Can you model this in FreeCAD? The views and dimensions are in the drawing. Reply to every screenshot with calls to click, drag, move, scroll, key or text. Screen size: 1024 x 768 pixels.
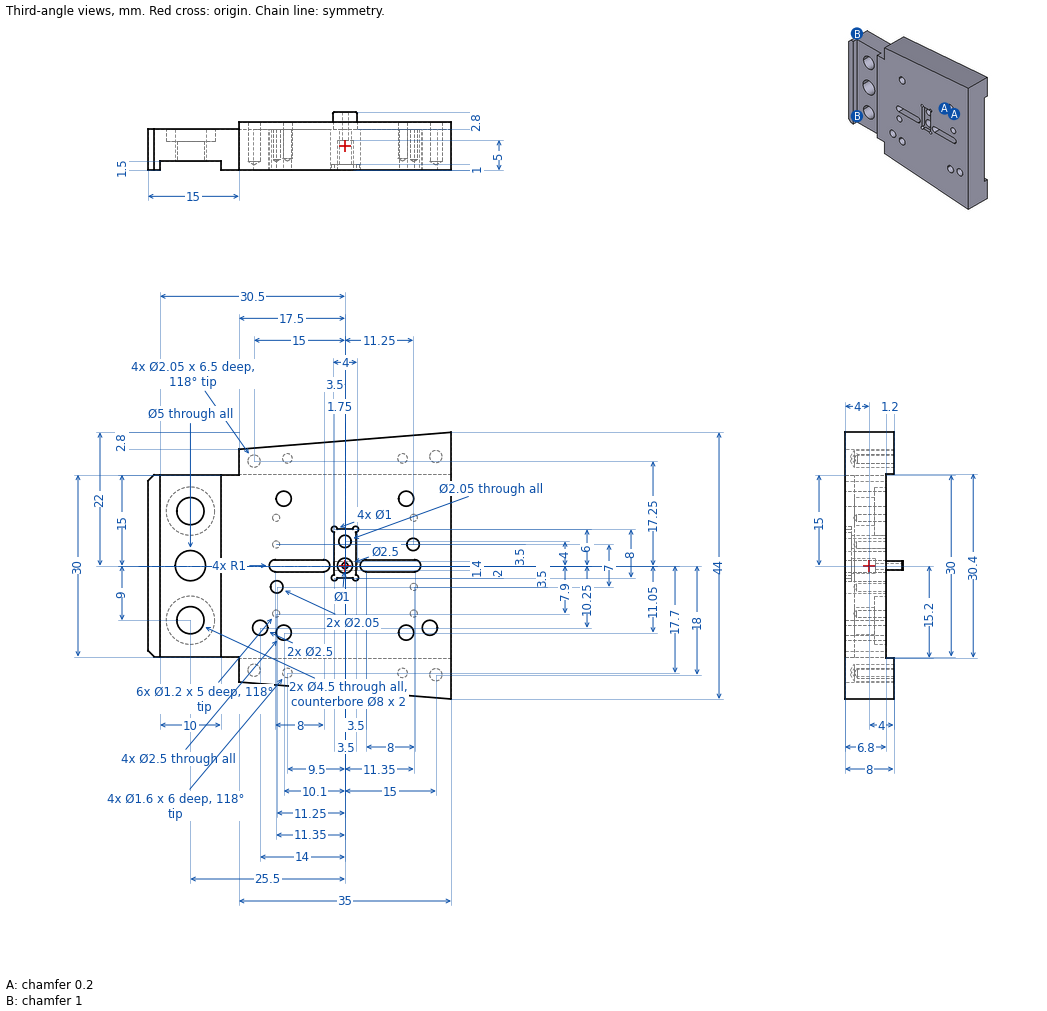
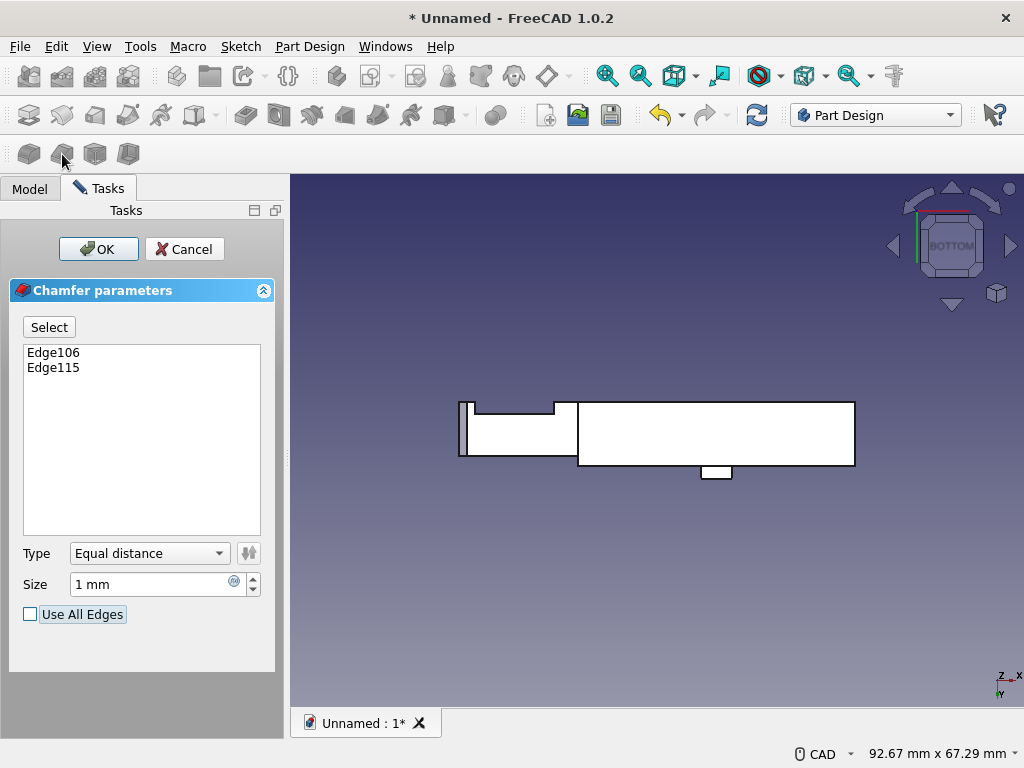
click(99, 249)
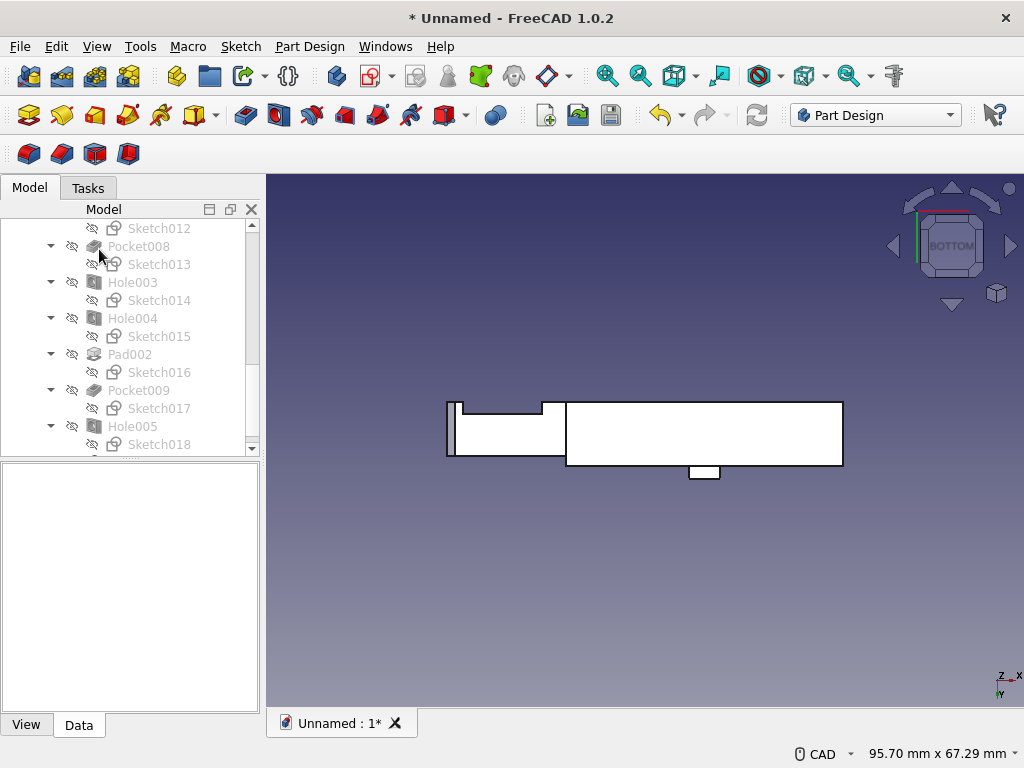
key(4)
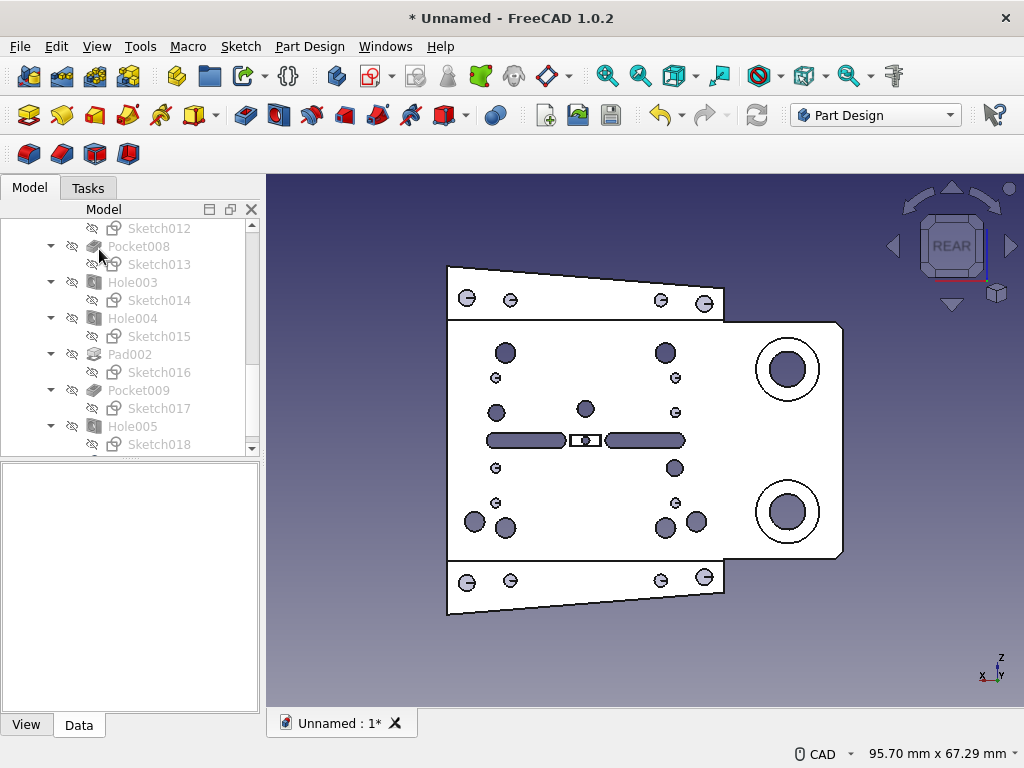
click(588, 508)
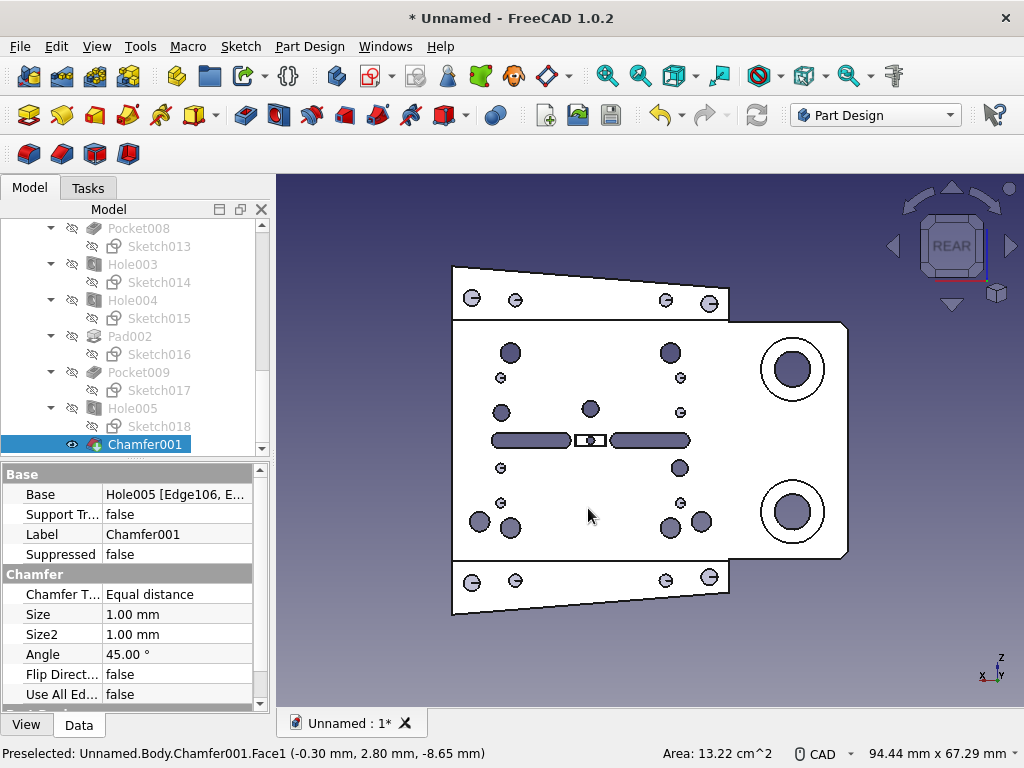
click(370, 76)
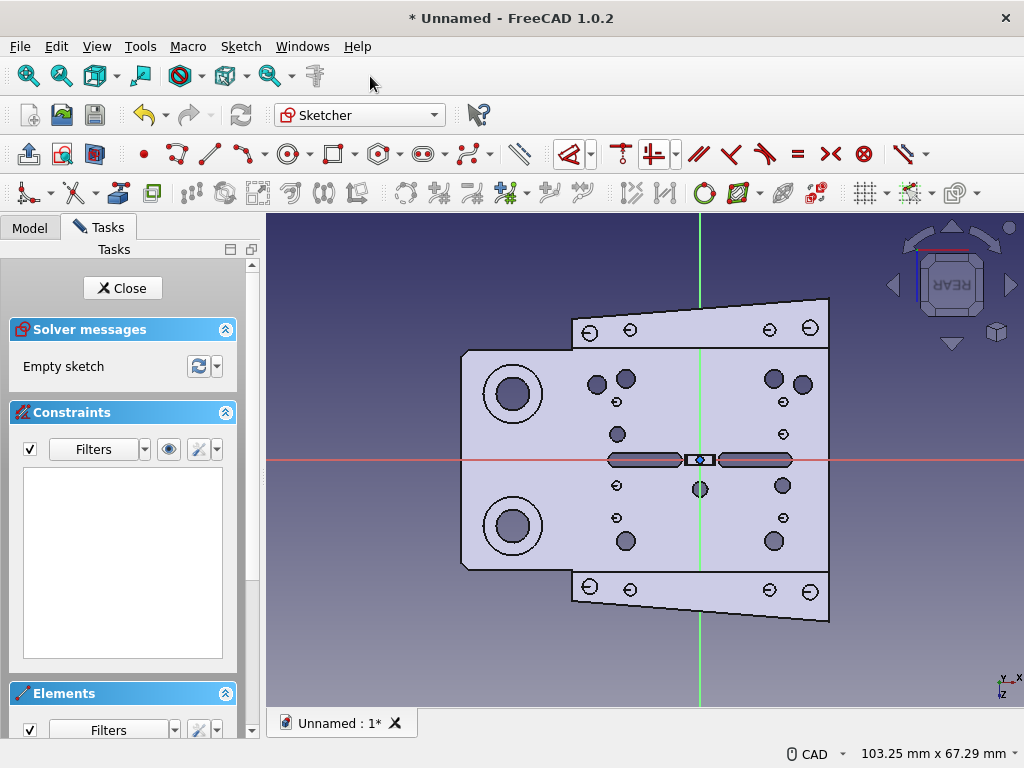
click(95, 154)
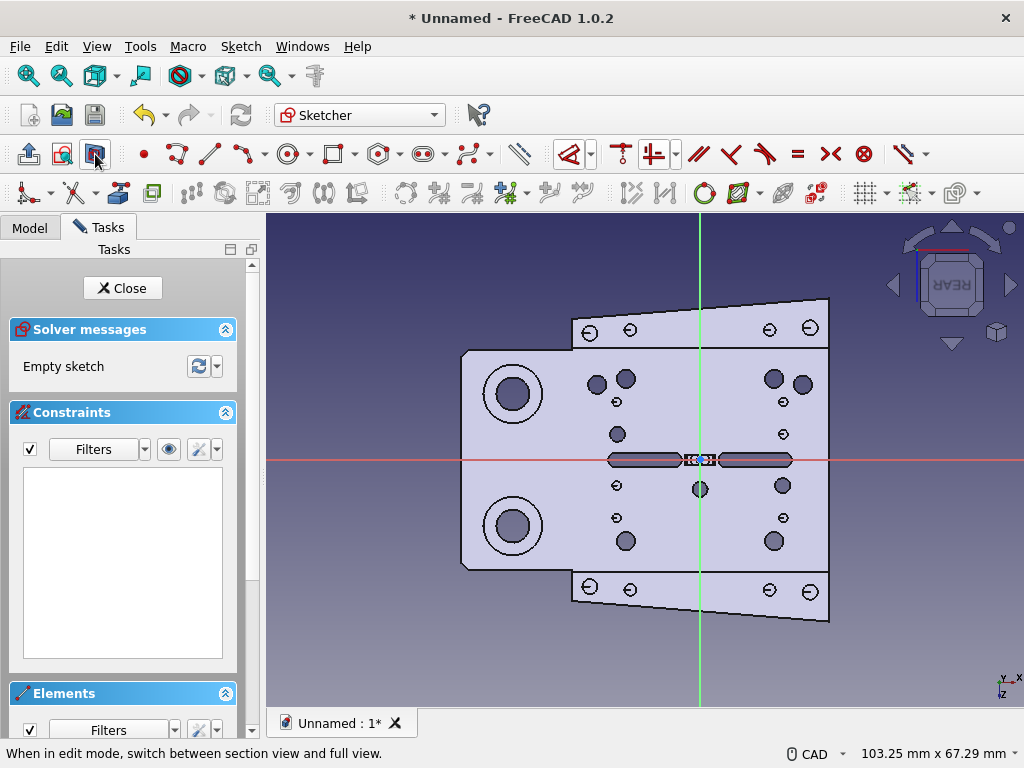
scroll(505, 460, up, 11)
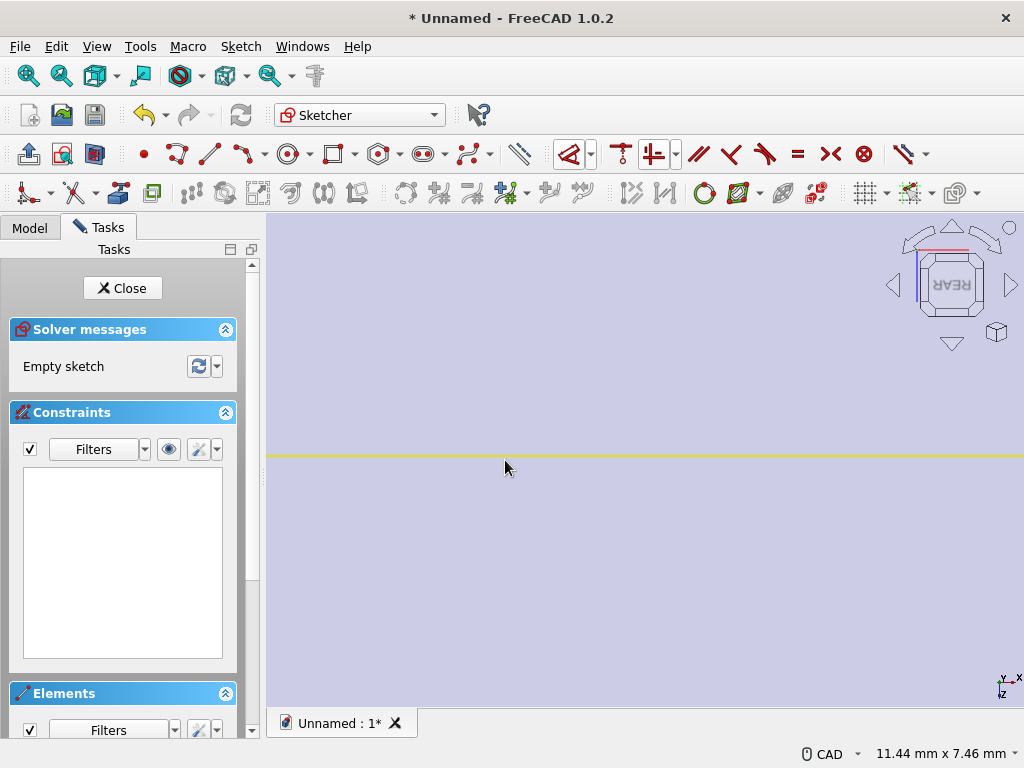
click(288, 154)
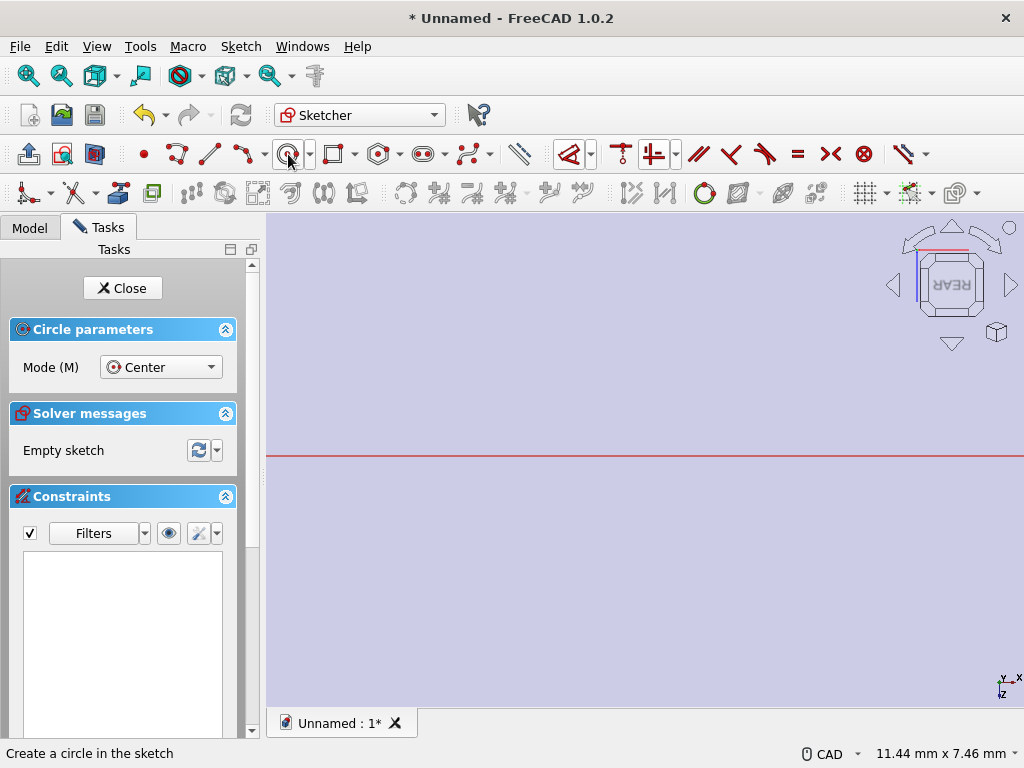
click(573, 456)
move(691, 339)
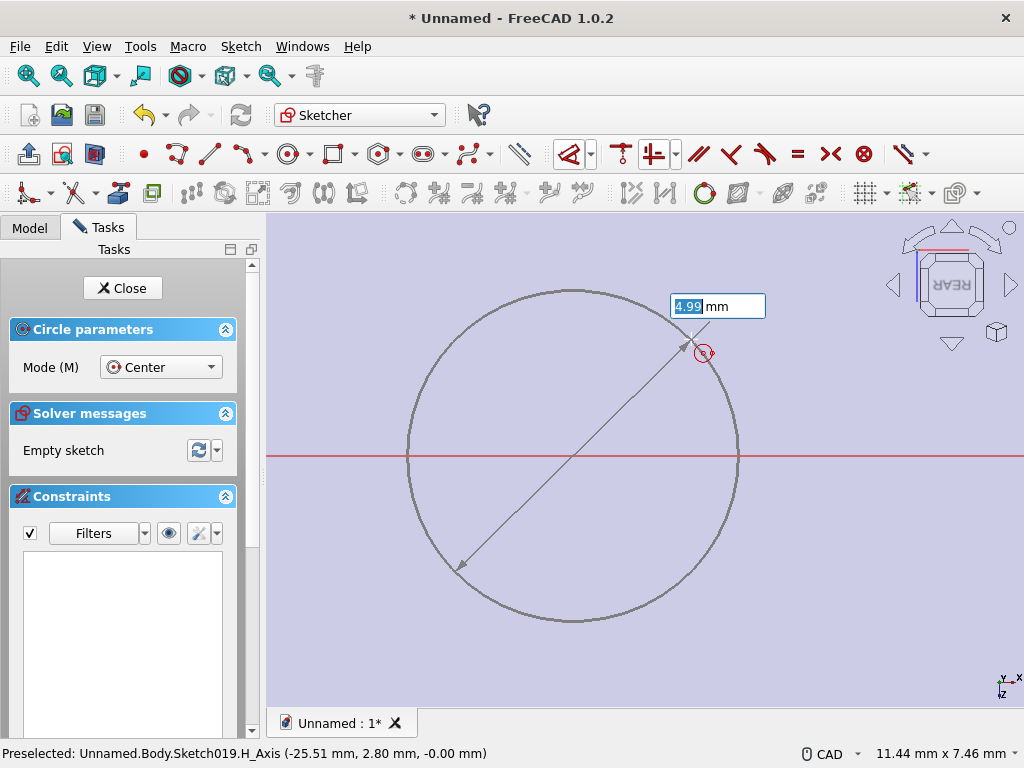
text(5)
key(Return)
key(Escape)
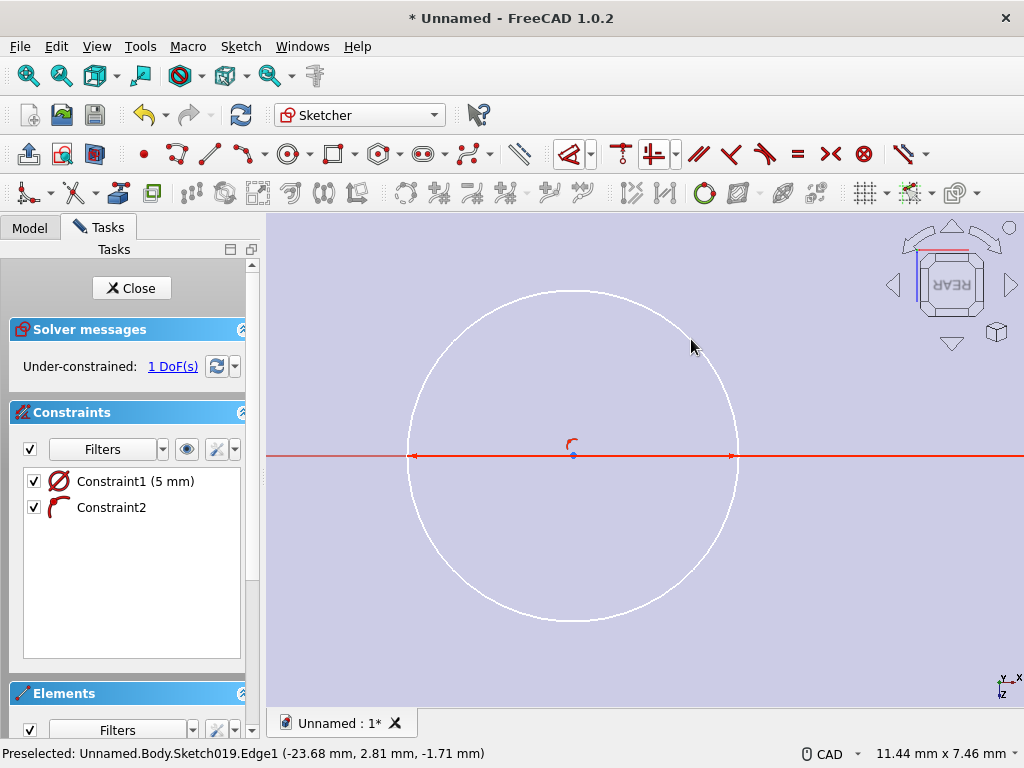
click(573, 456)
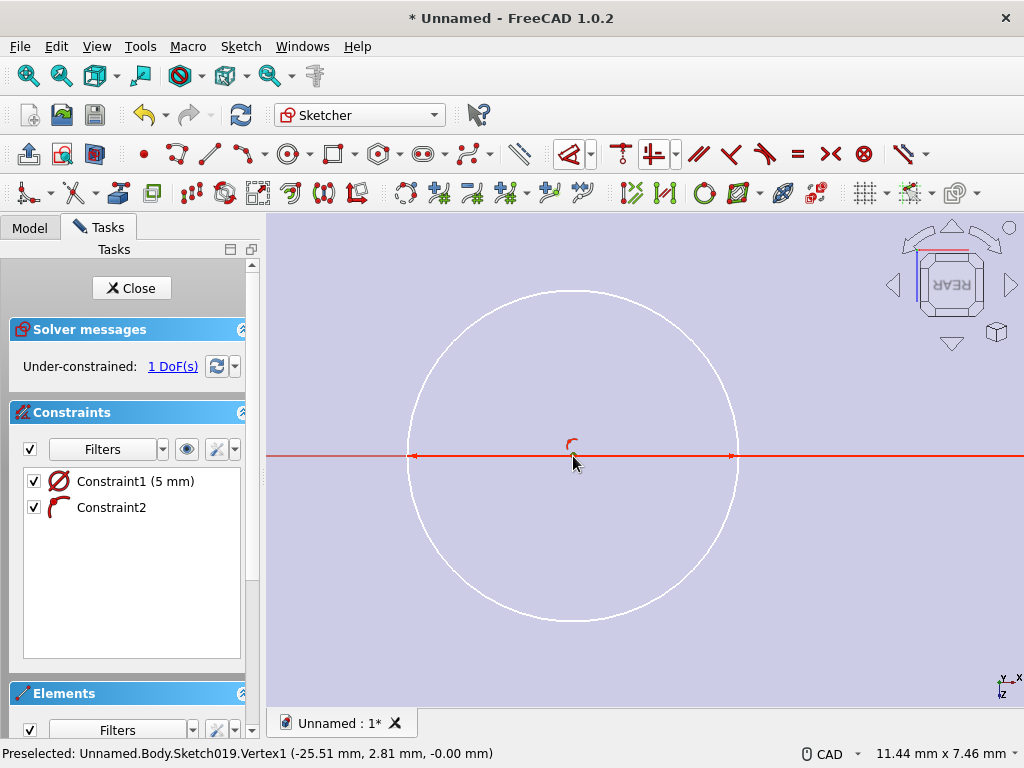
click(590, 154)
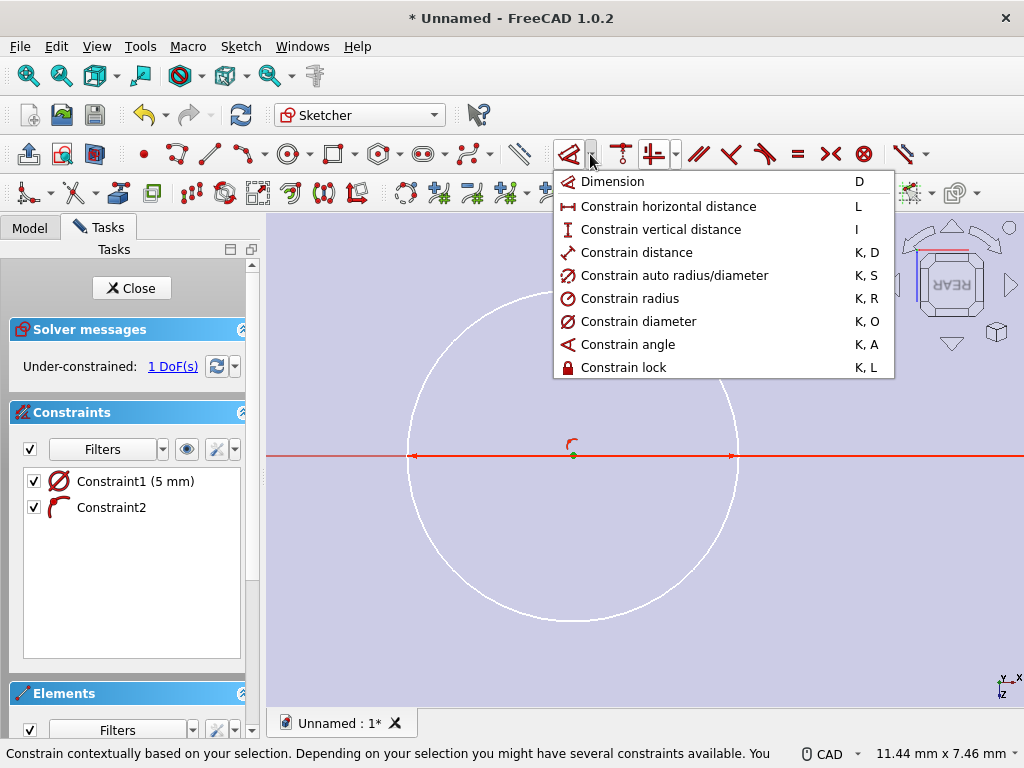
click(724, 206)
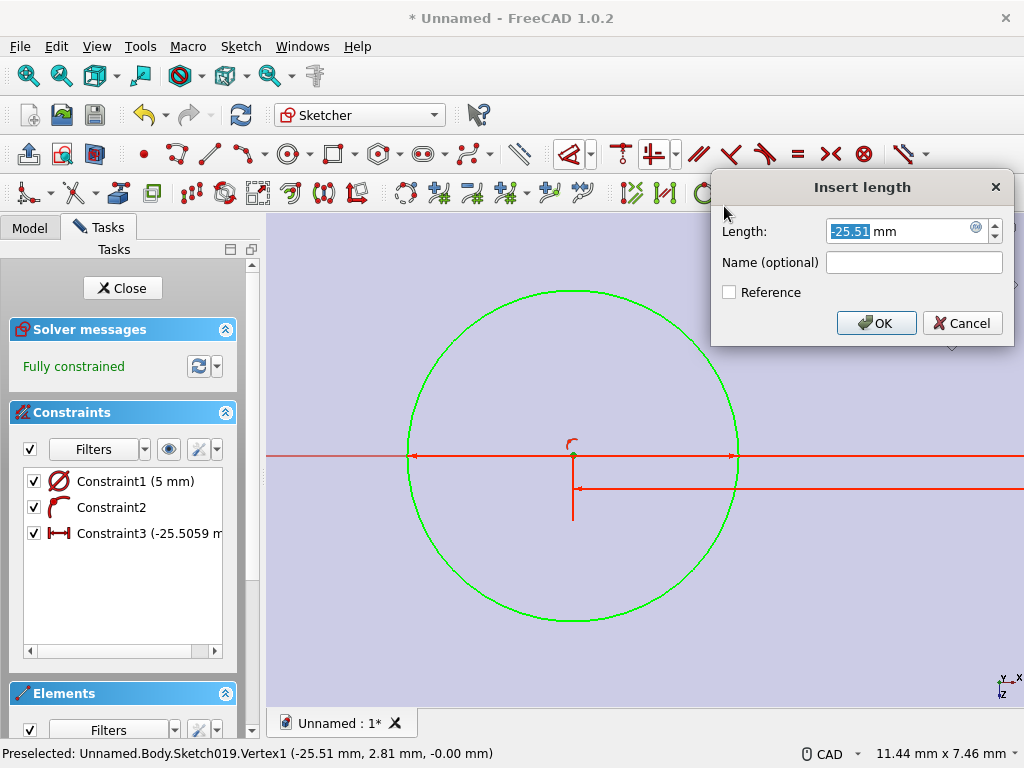
text(-25.5)
key(Return)